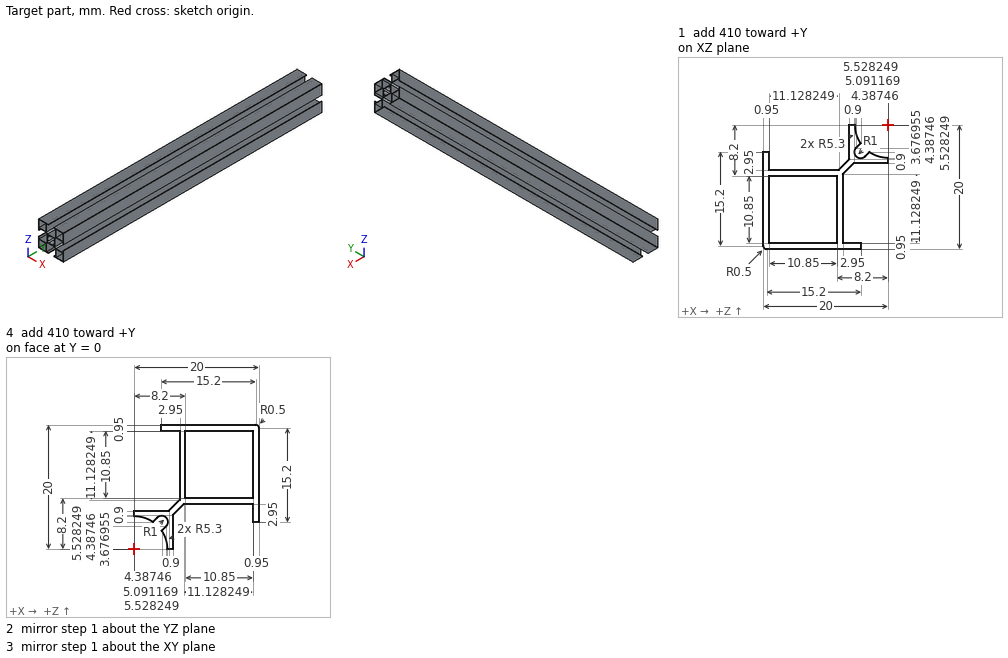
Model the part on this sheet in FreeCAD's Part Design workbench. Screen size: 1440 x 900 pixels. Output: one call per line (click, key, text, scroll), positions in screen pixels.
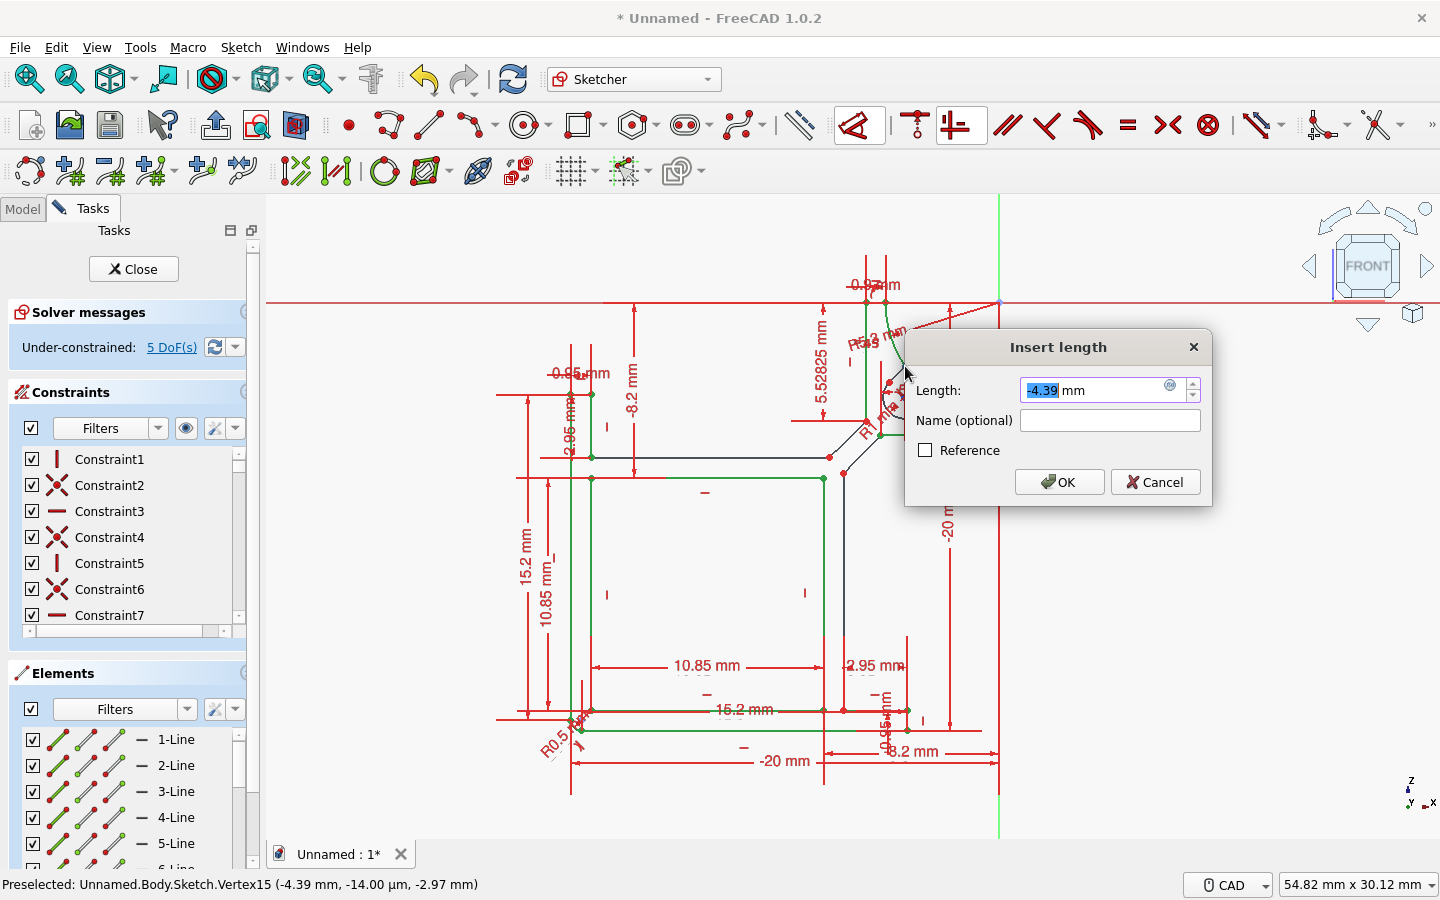
text(-4.38746)
key(Return)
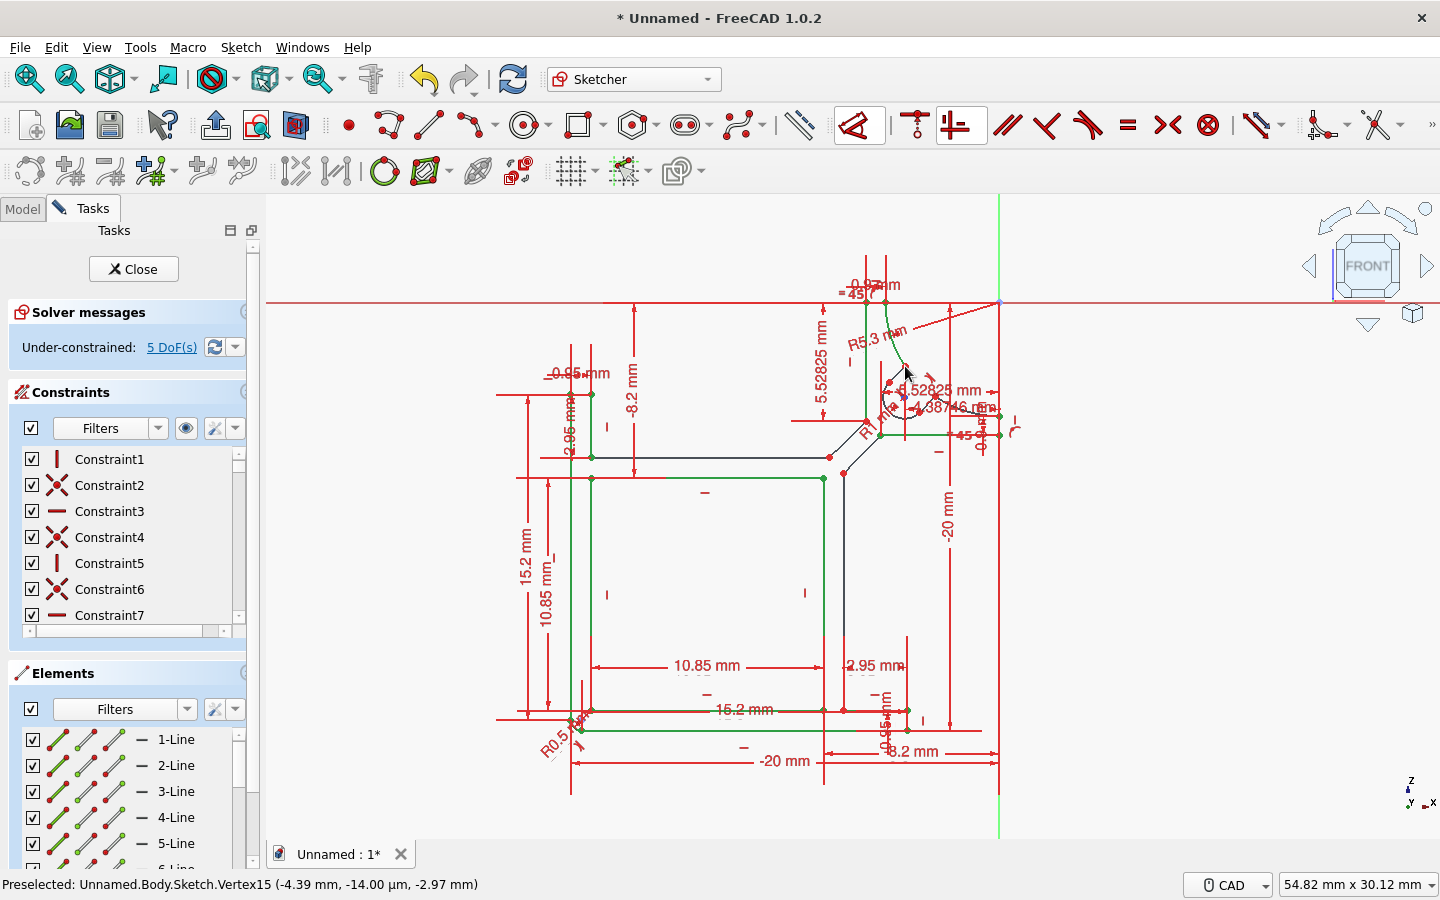
click(935, 396)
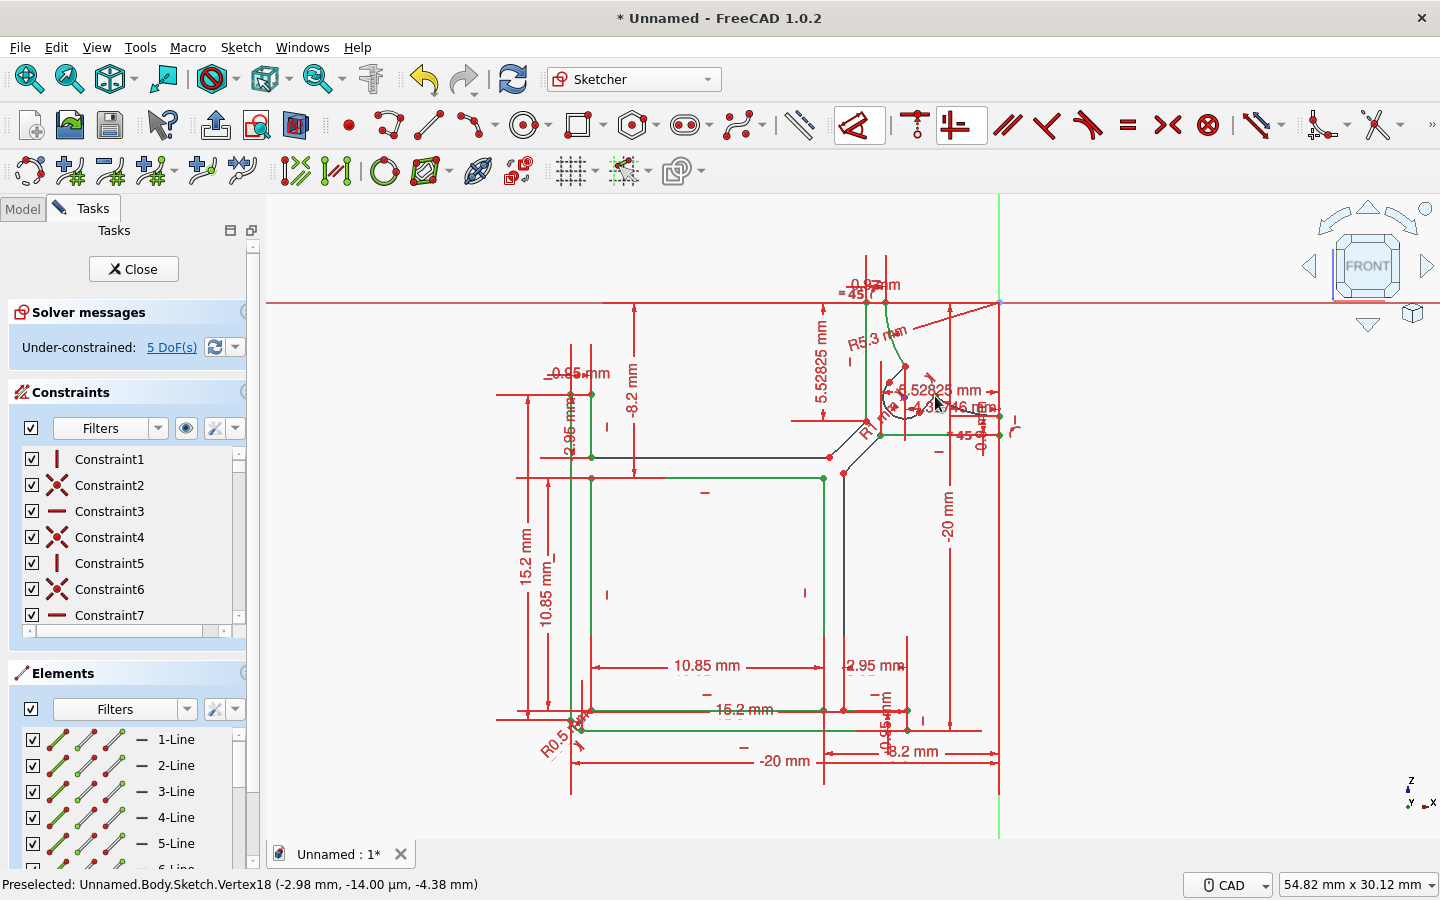
click(880, 126)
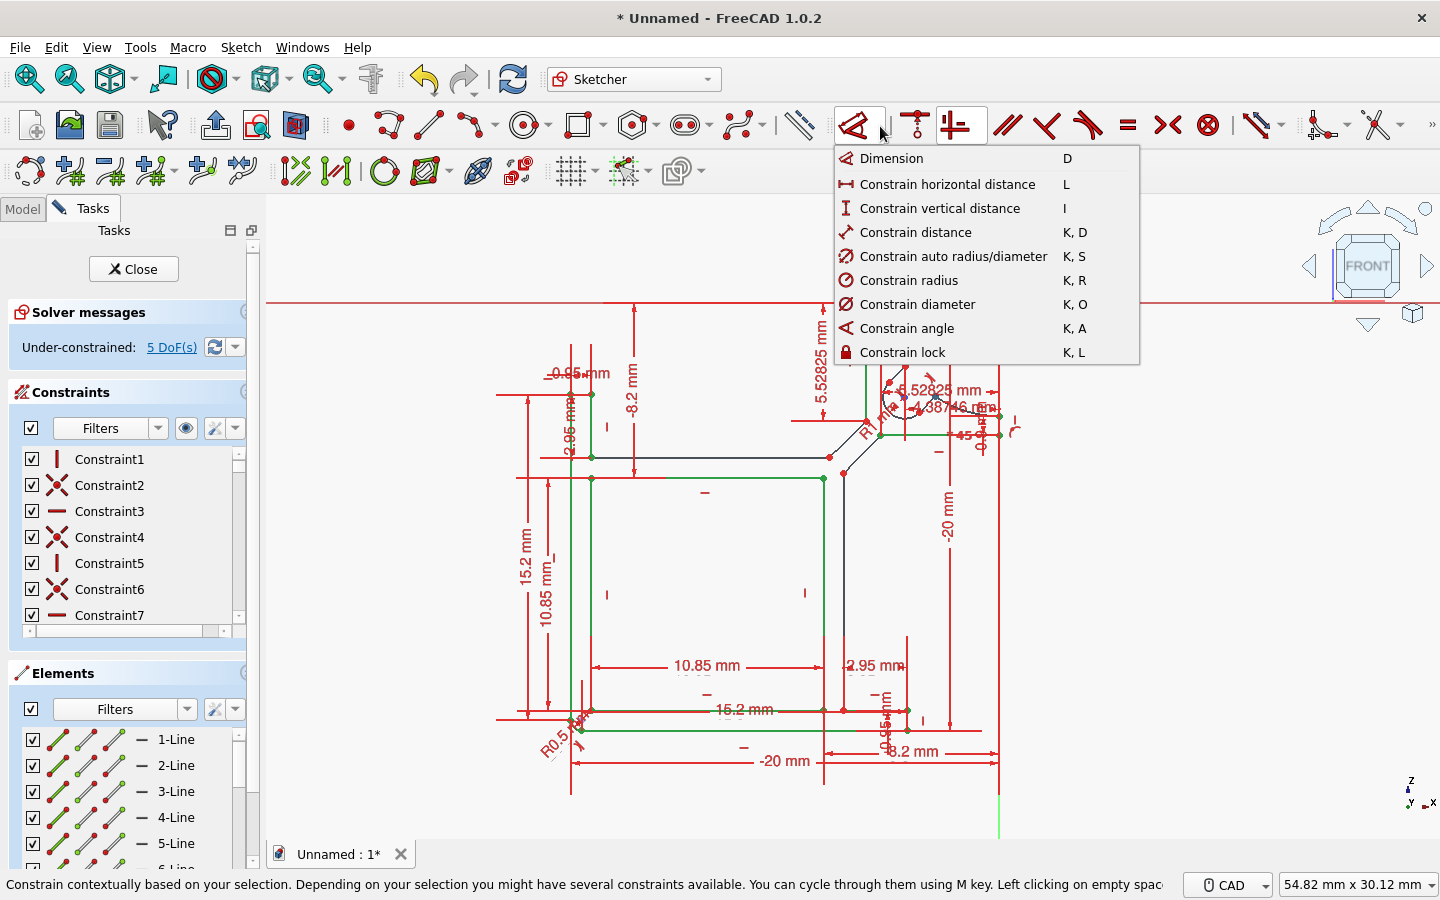
click(987, 208)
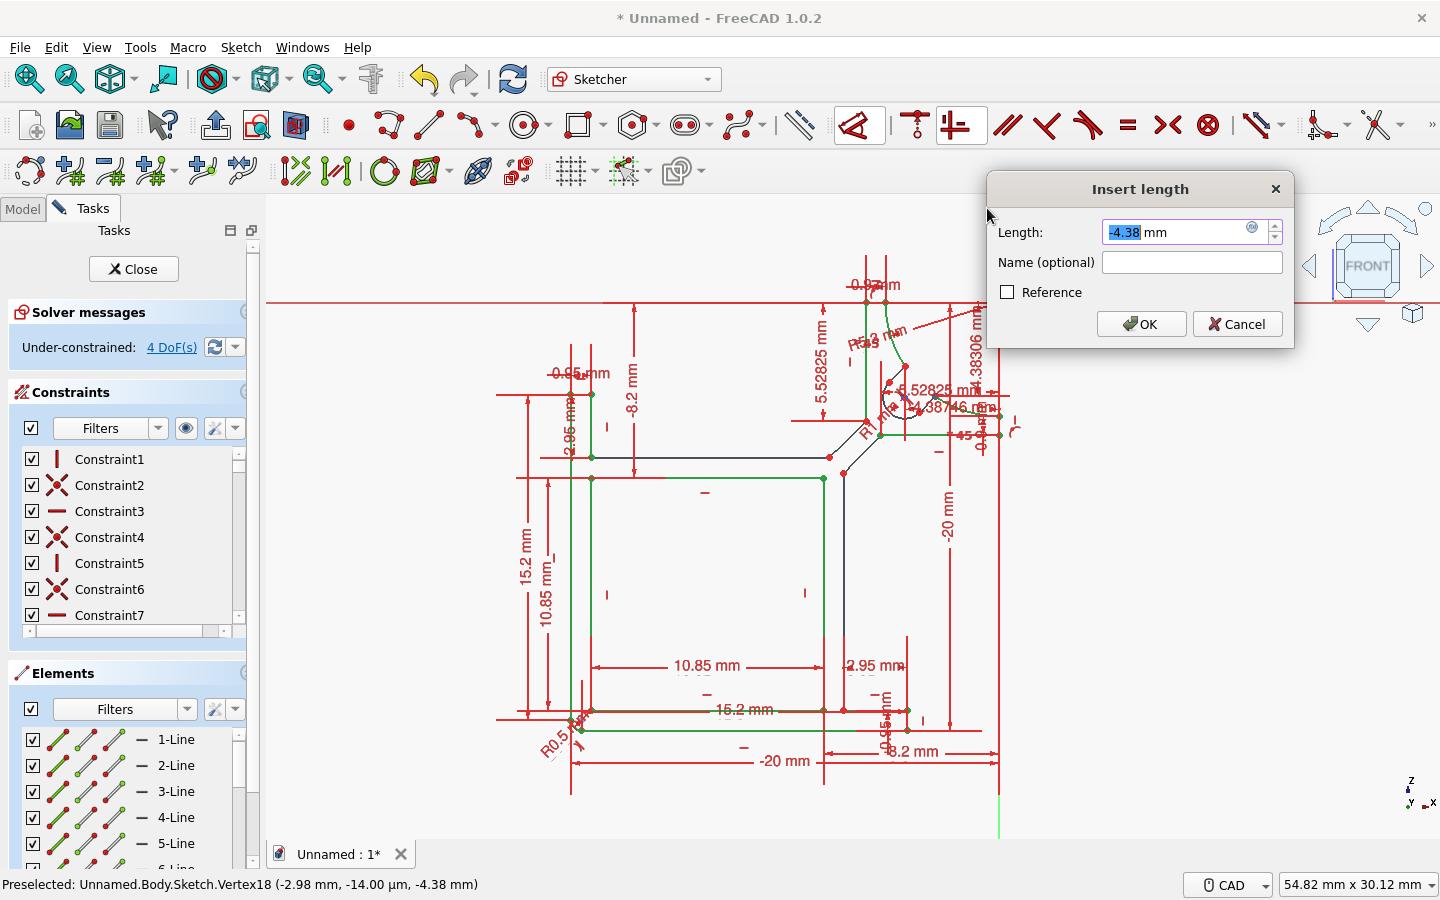
text(-4.38746)
key(Return)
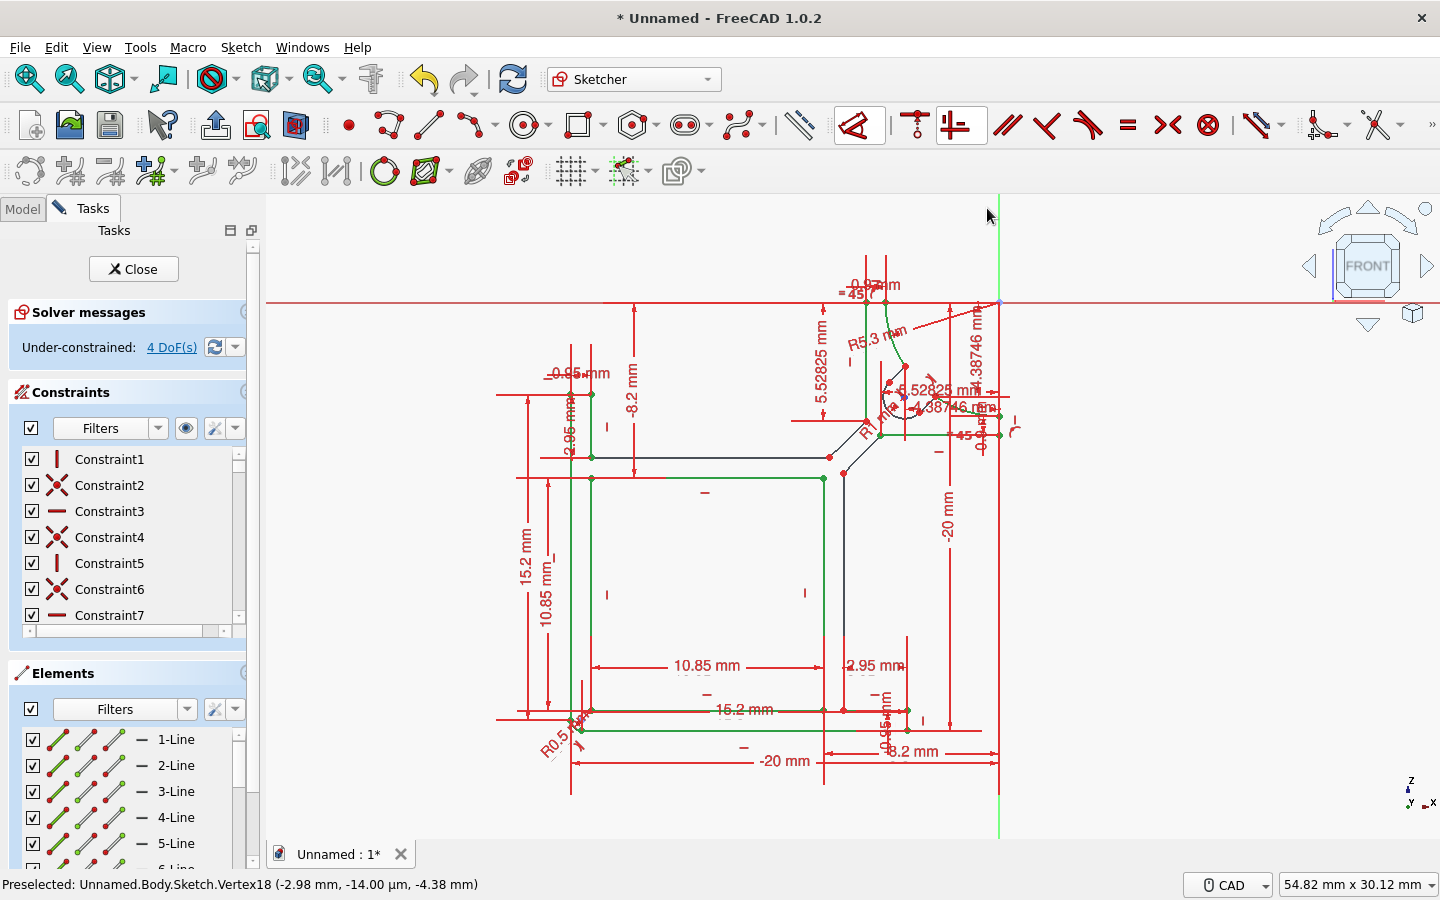
click(663, 458)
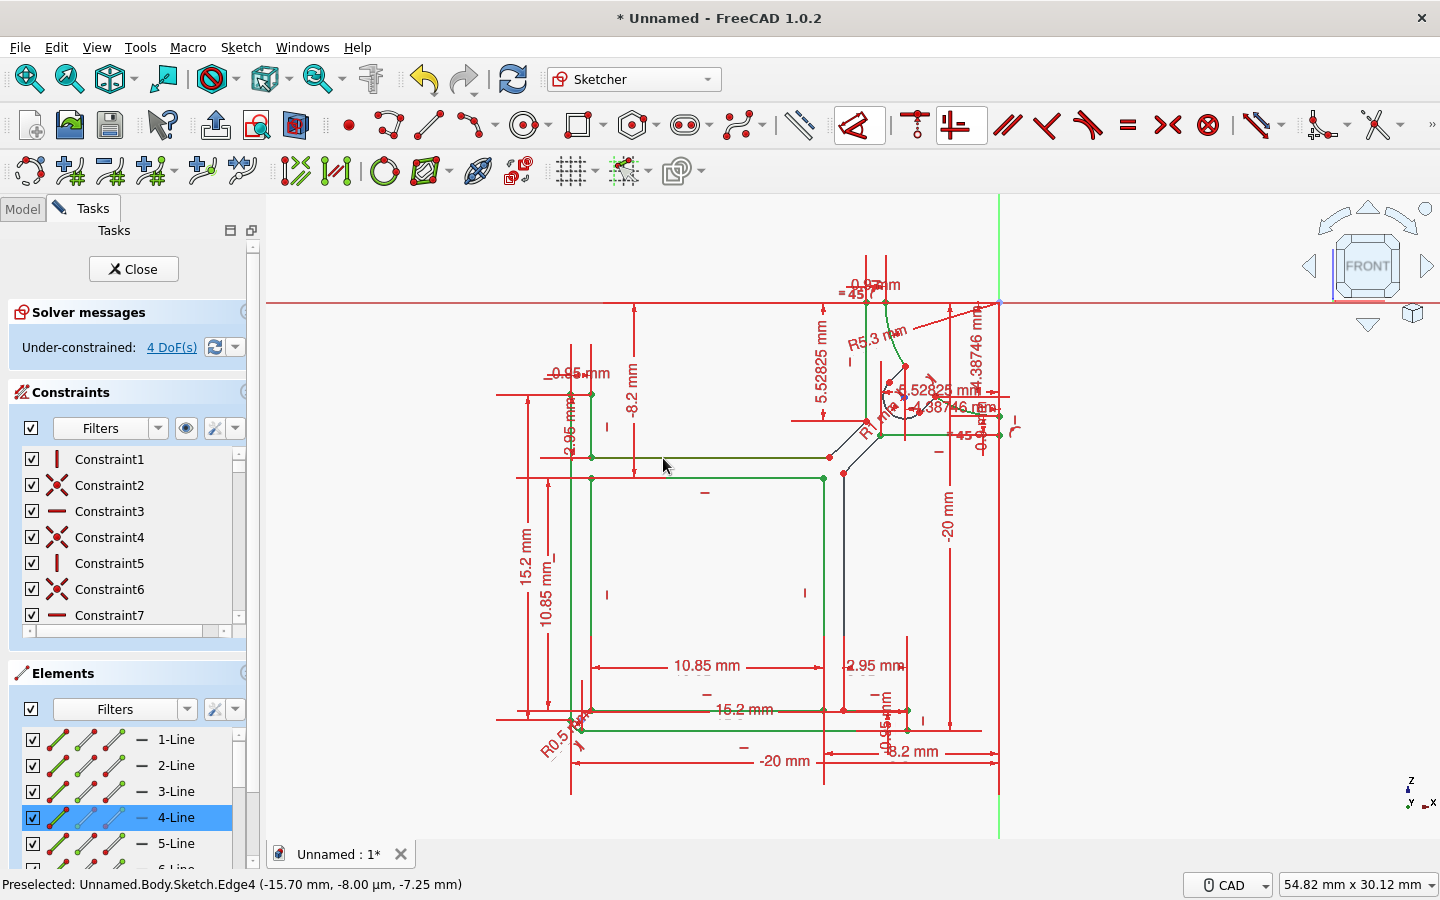
key(l)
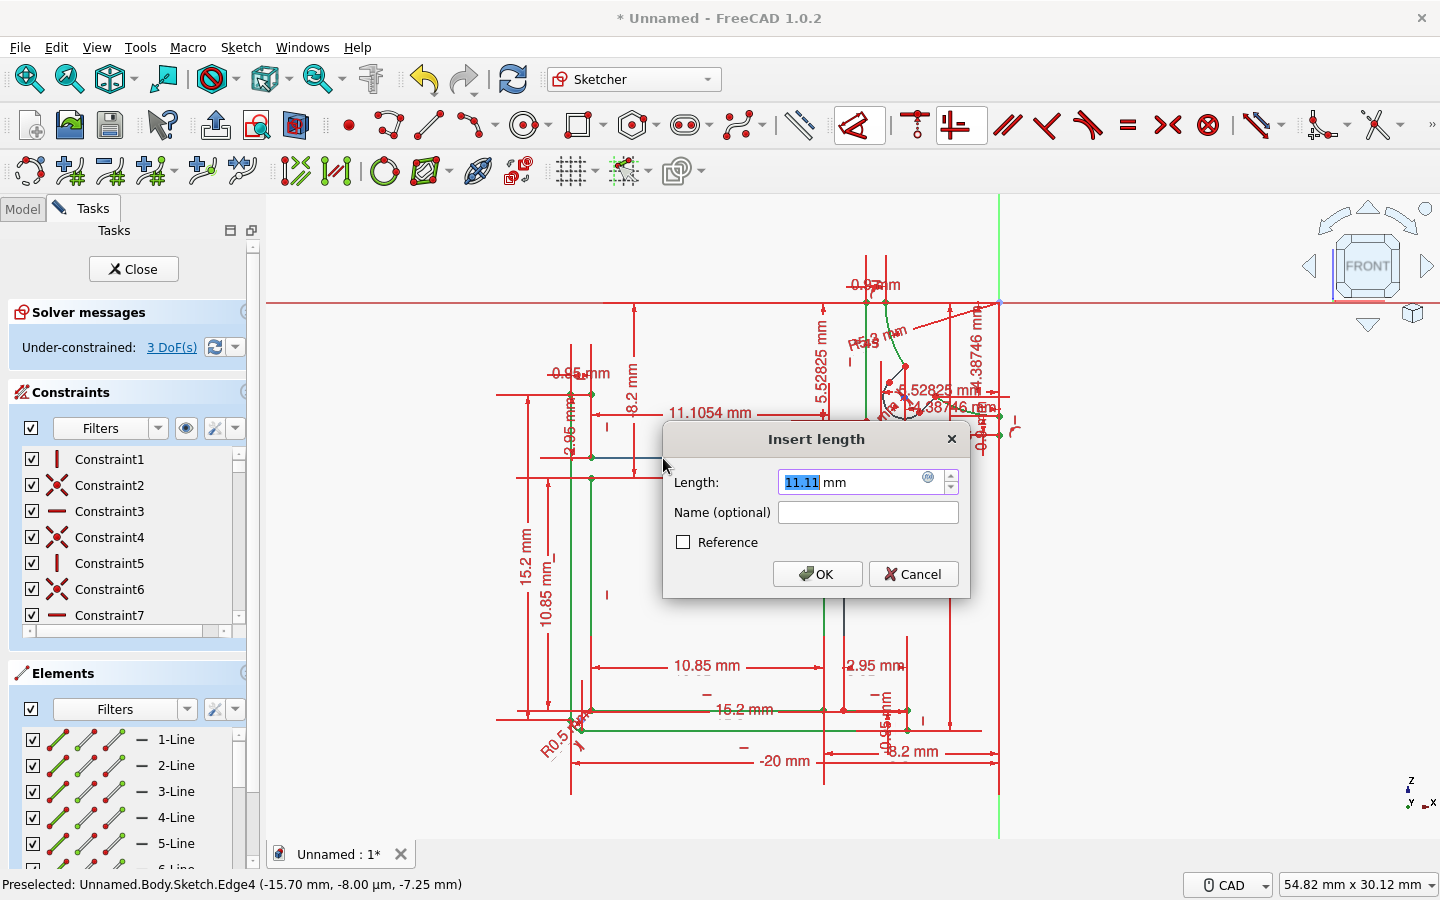
text(11.128249)
key(Return)